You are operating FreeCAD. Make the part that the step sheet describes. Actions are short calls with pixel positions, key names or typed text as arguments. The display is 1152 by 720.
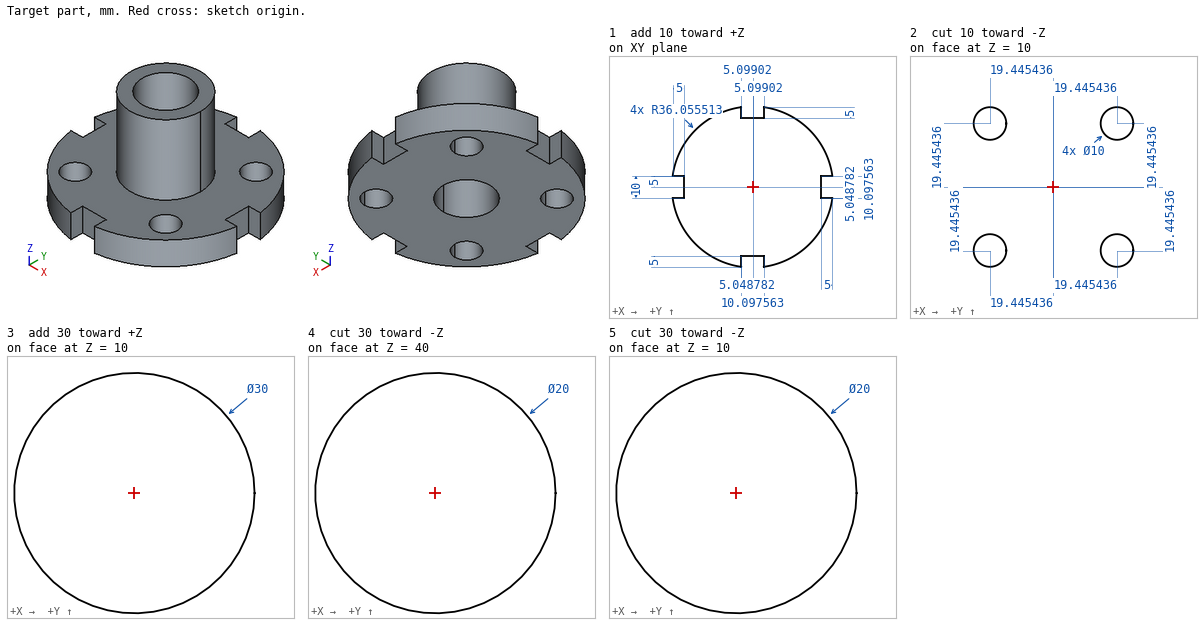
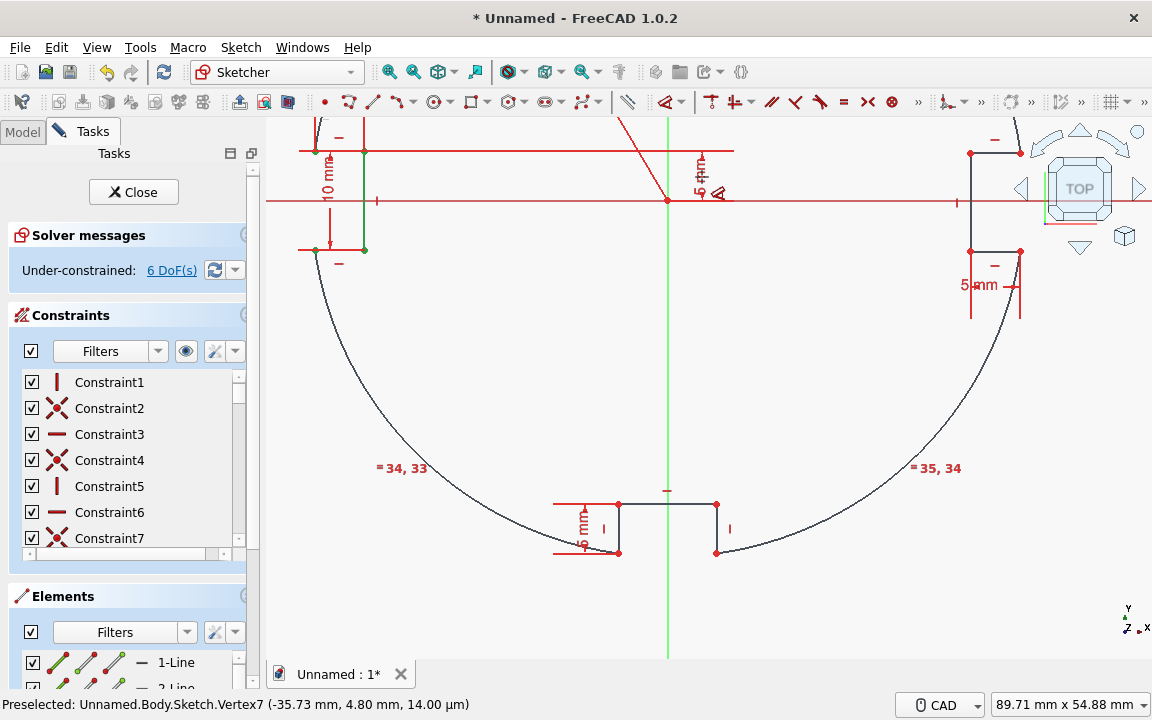
scroll(618, 541, down, 4)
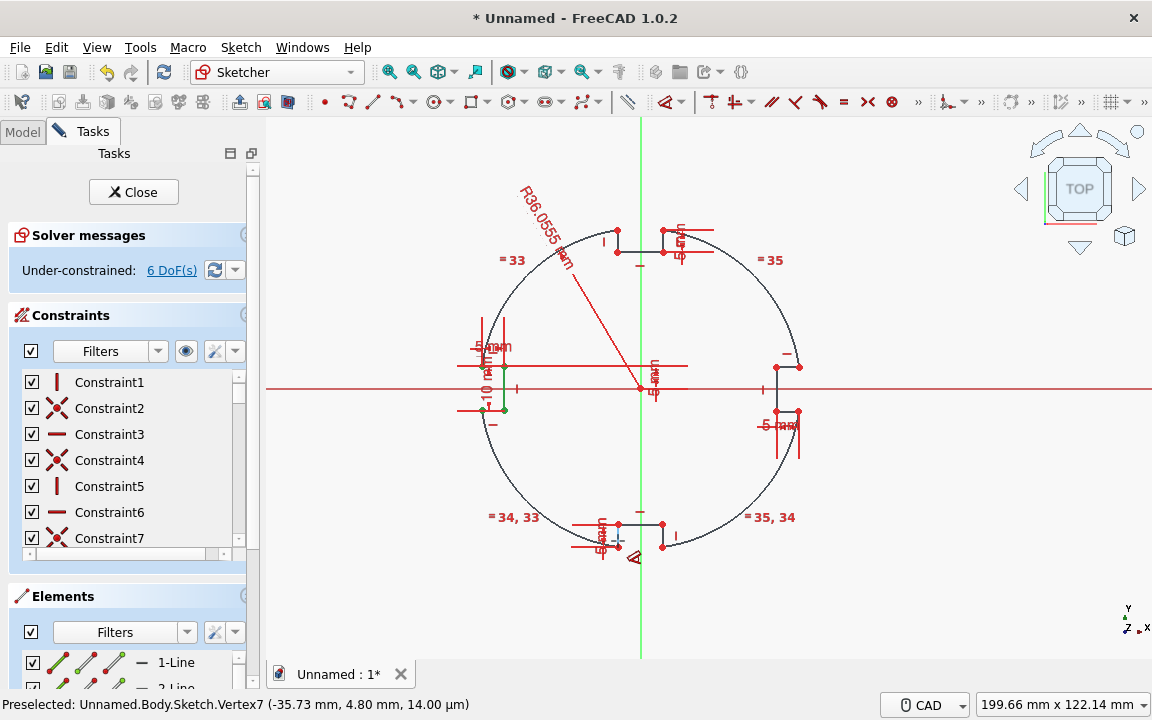
scroll(663, 230, up, 3)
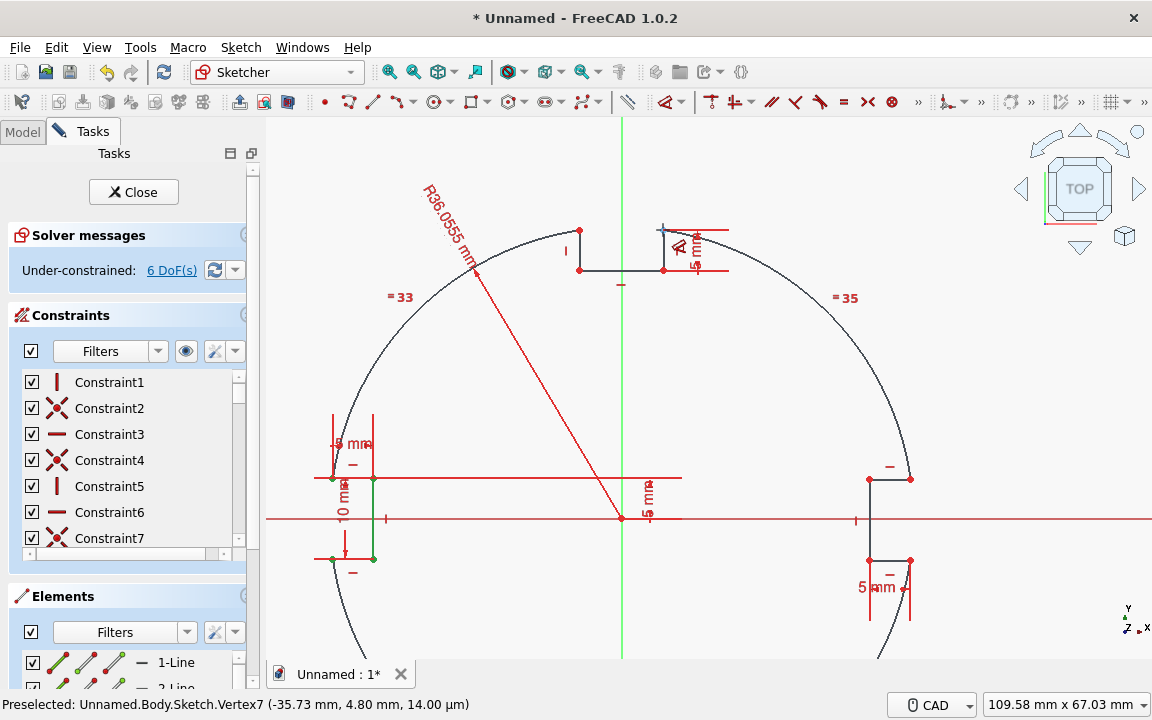
click(664, 230)
click(643, 196)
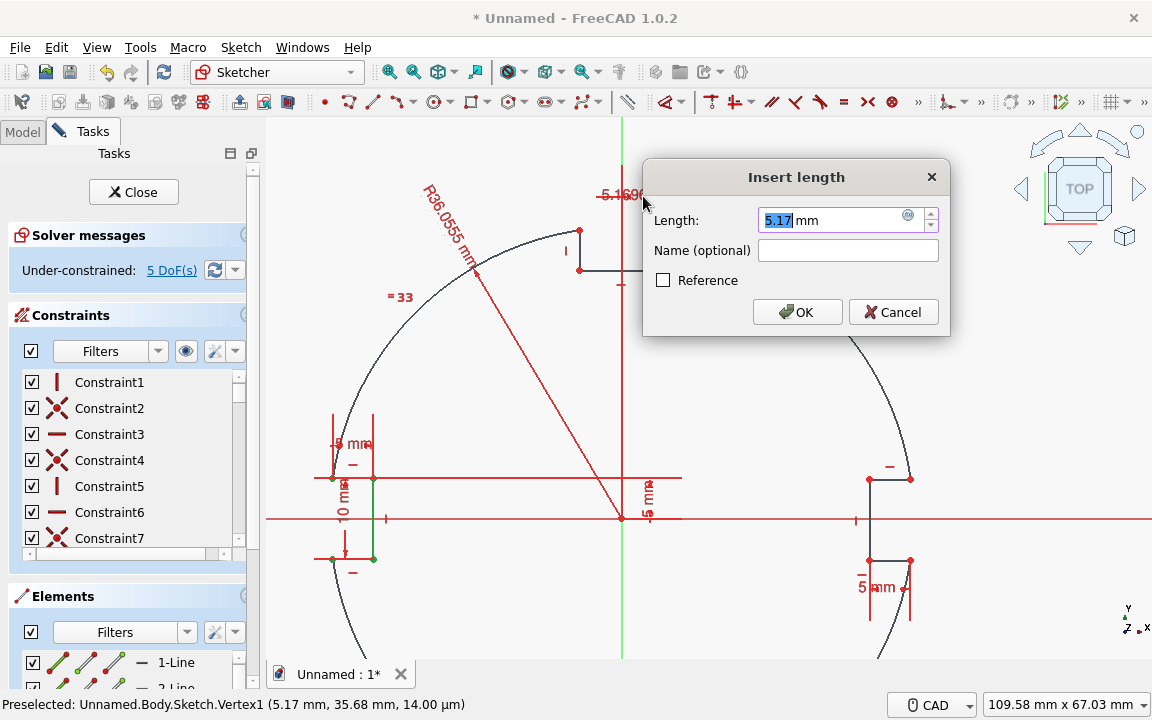
text(5.09902)
key(Return)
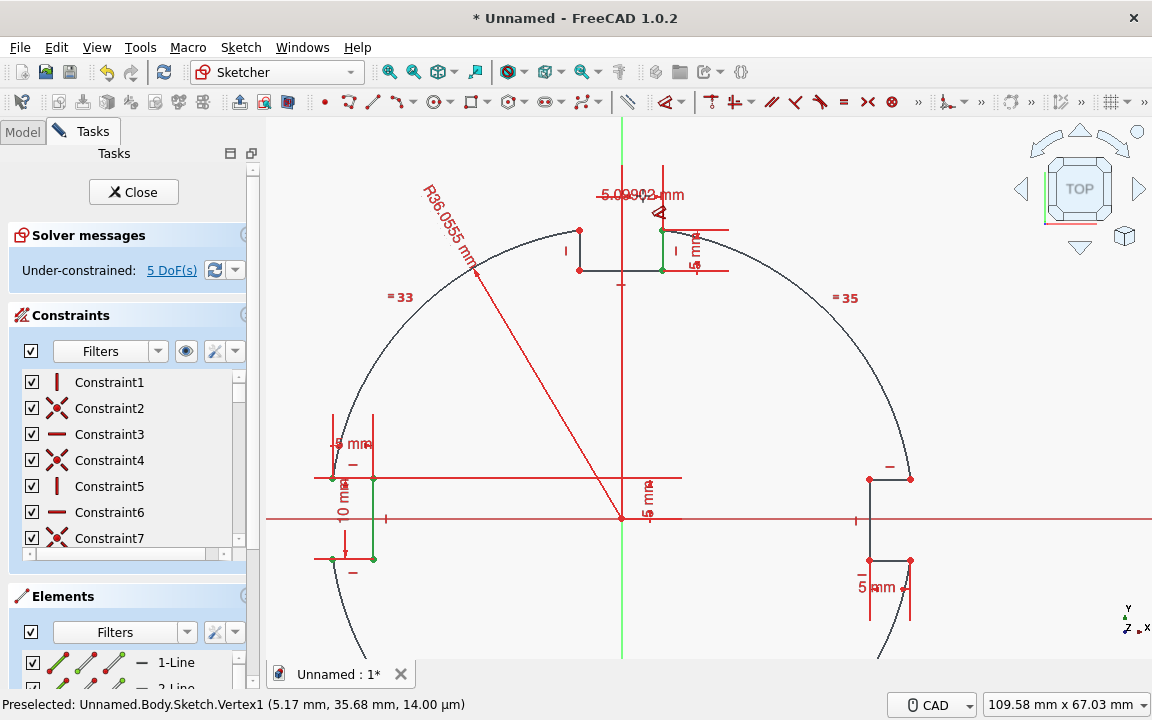
click(580, 271)
click(601, 237)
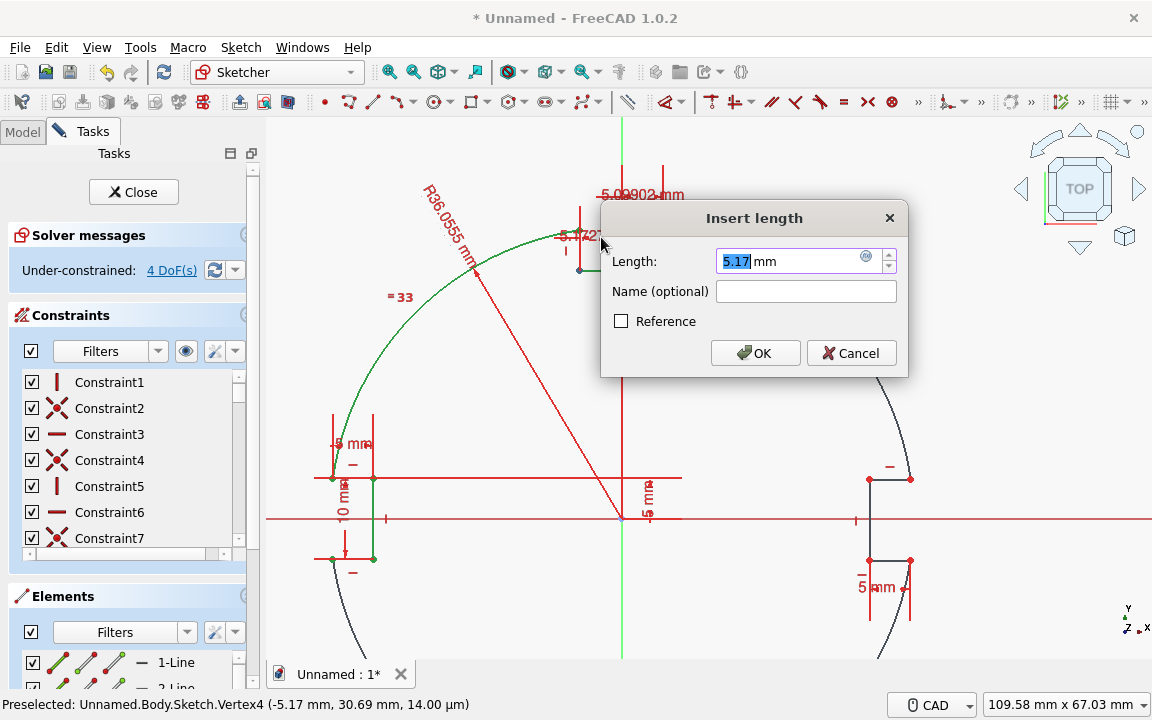
text(5.09902)
key(Return)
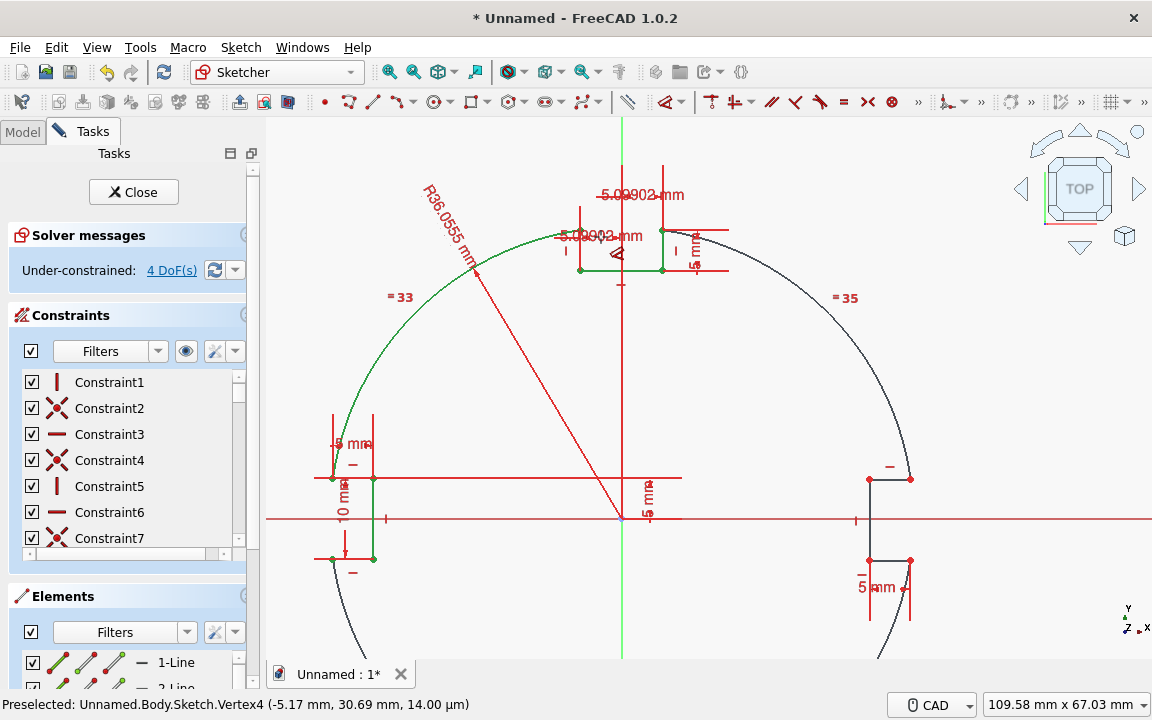
scroll(663, 229, down, 3)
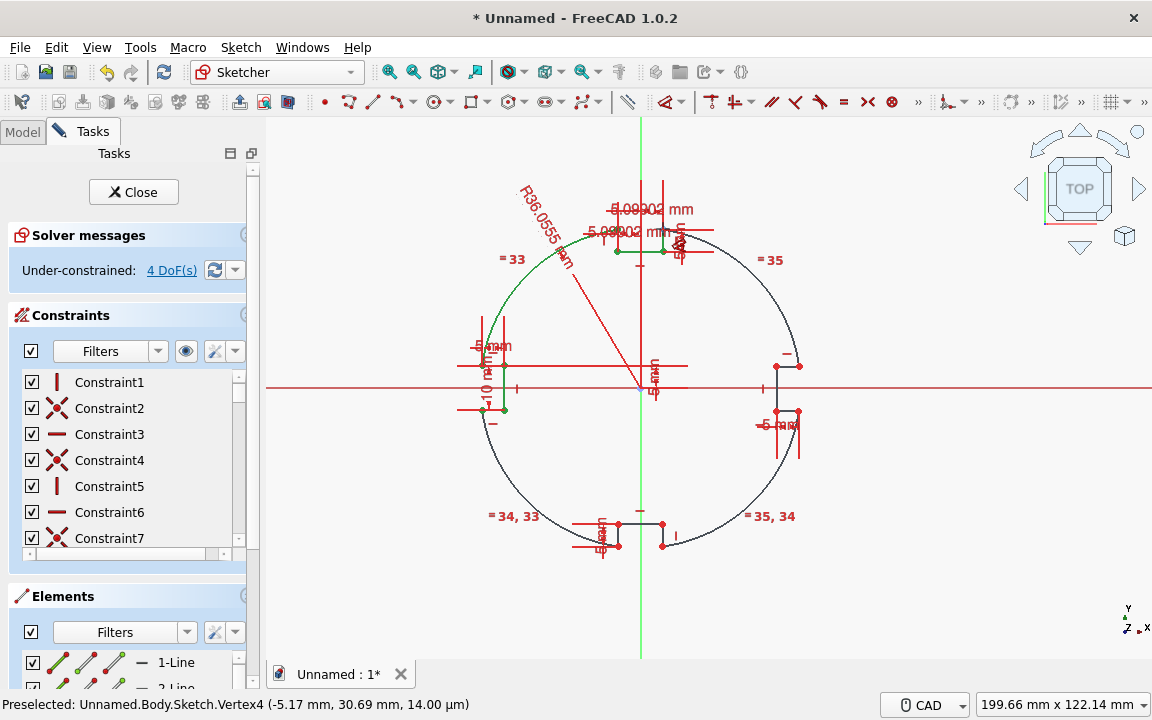
scroll(632, 524, up, 3)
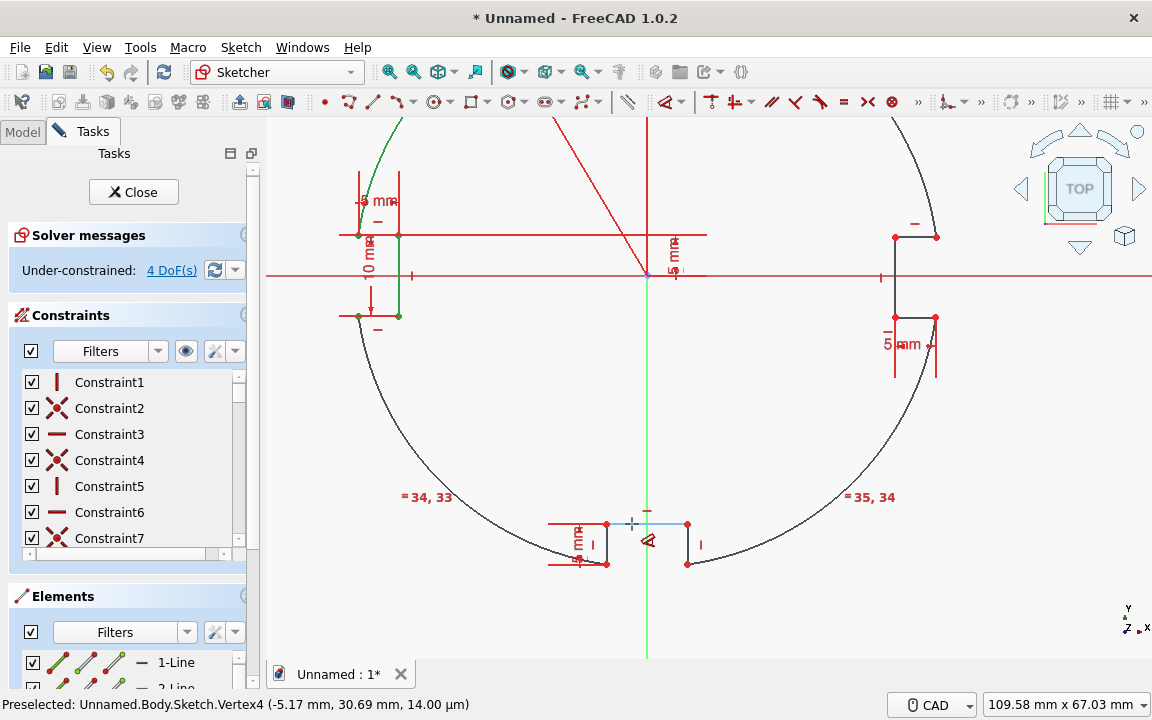
click(631, 524)
click(666, 558)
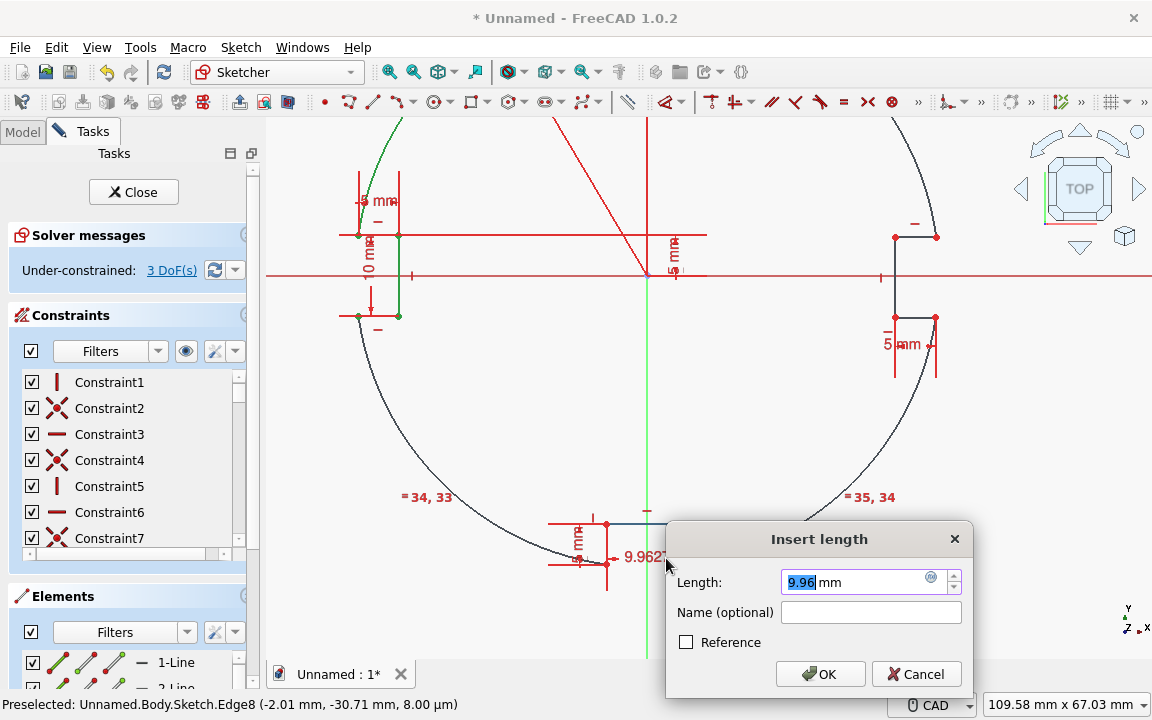
text(10.097563)
key(Return)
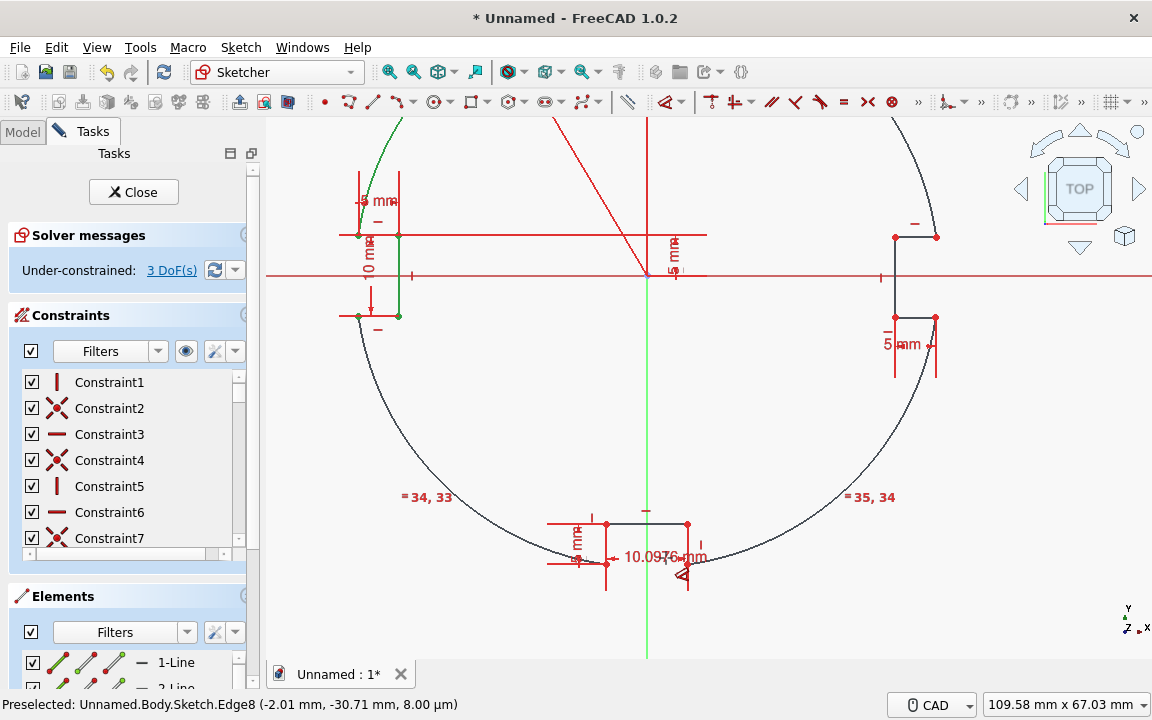
click(895, 293)
click(929, 259)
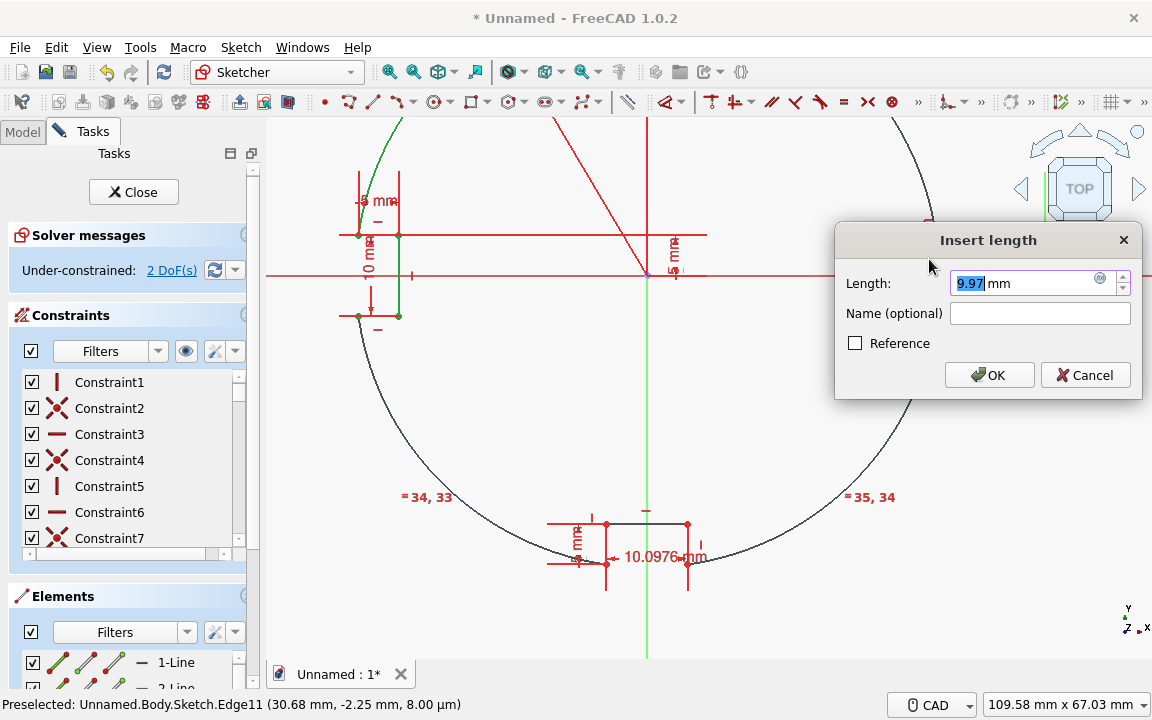
text(10.097563)
key(Return)